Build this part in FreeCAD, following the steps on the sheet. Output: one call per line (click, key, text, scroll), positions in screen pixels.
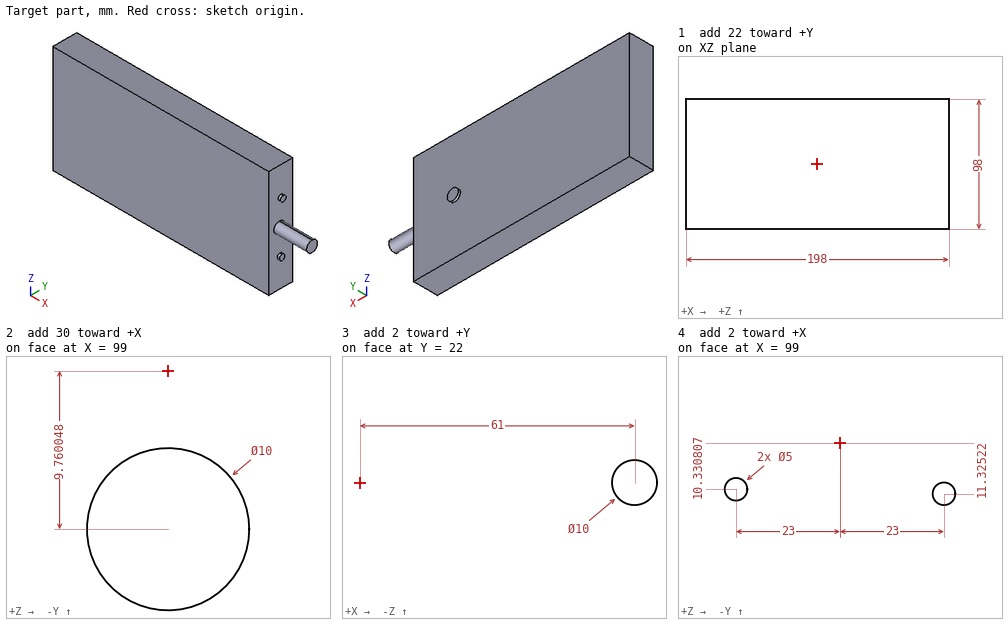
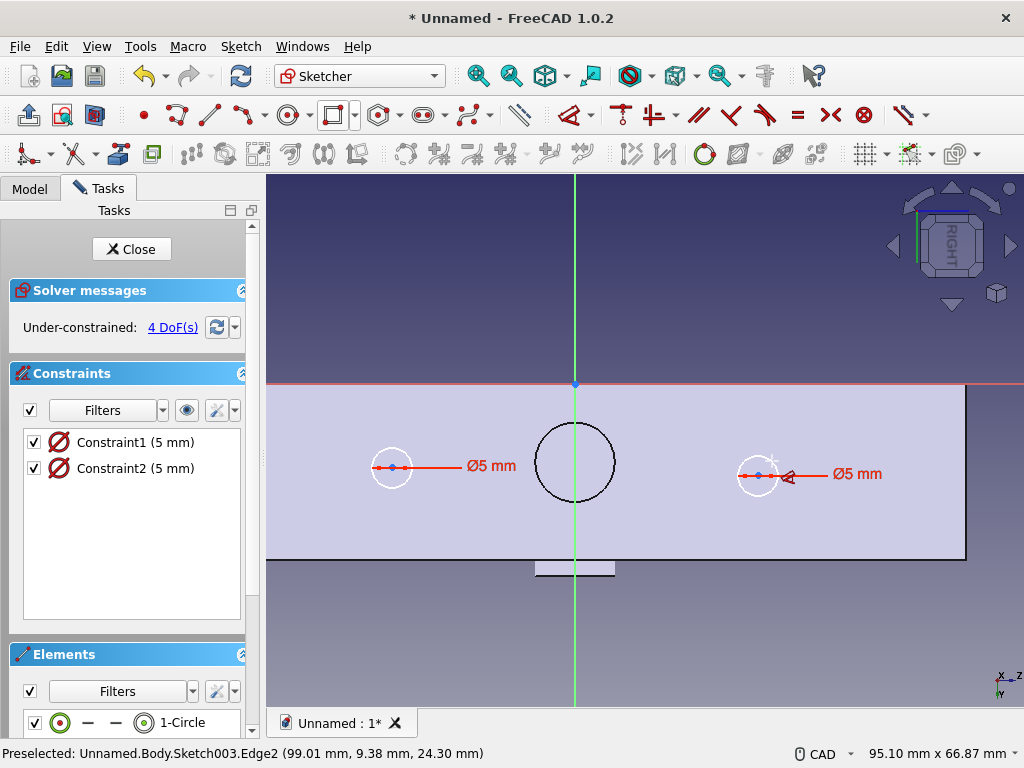
click(392, 468)
click(484, 350)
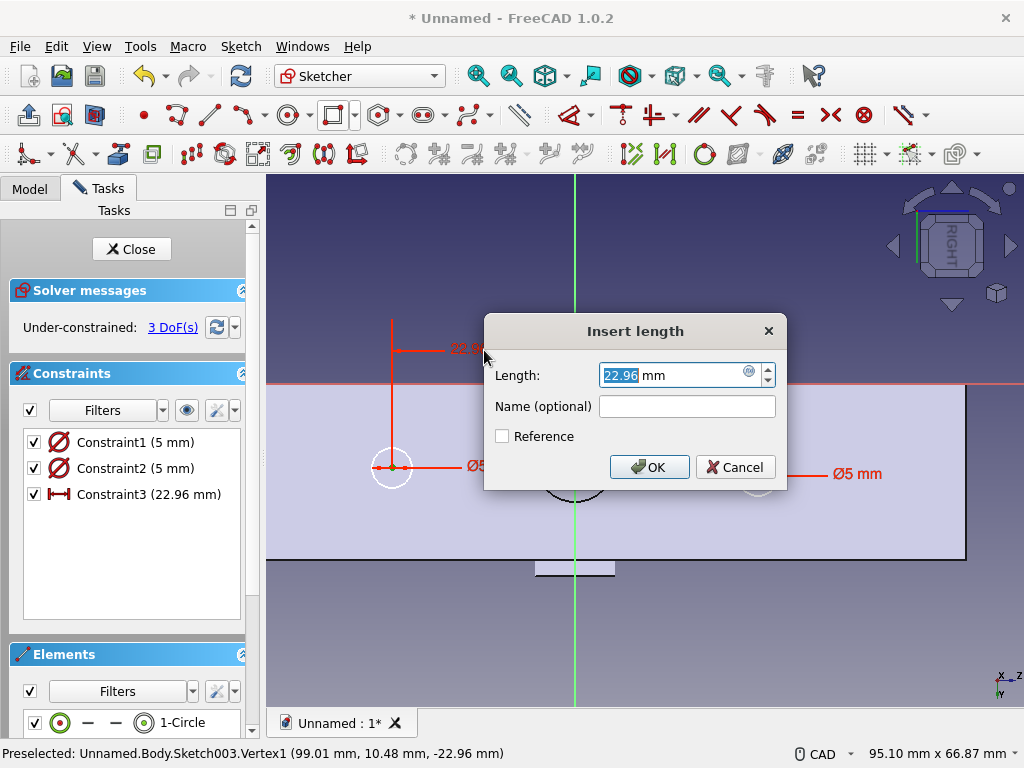
text(23)
key(Return)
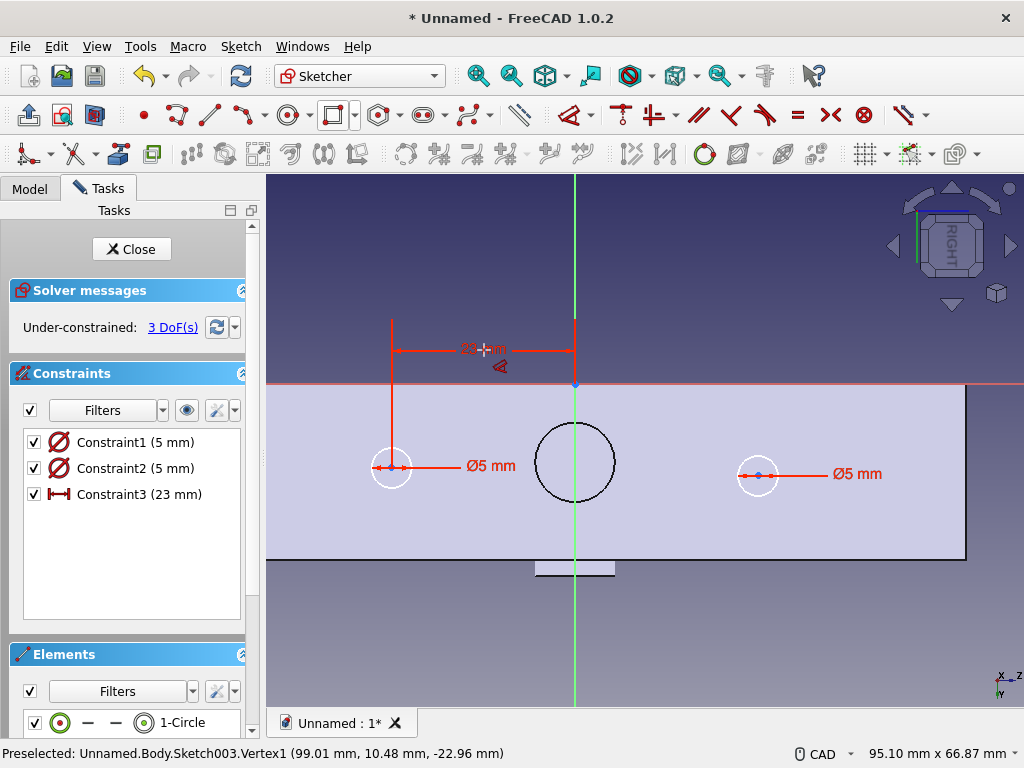
click(758, 476)
click(667, 350)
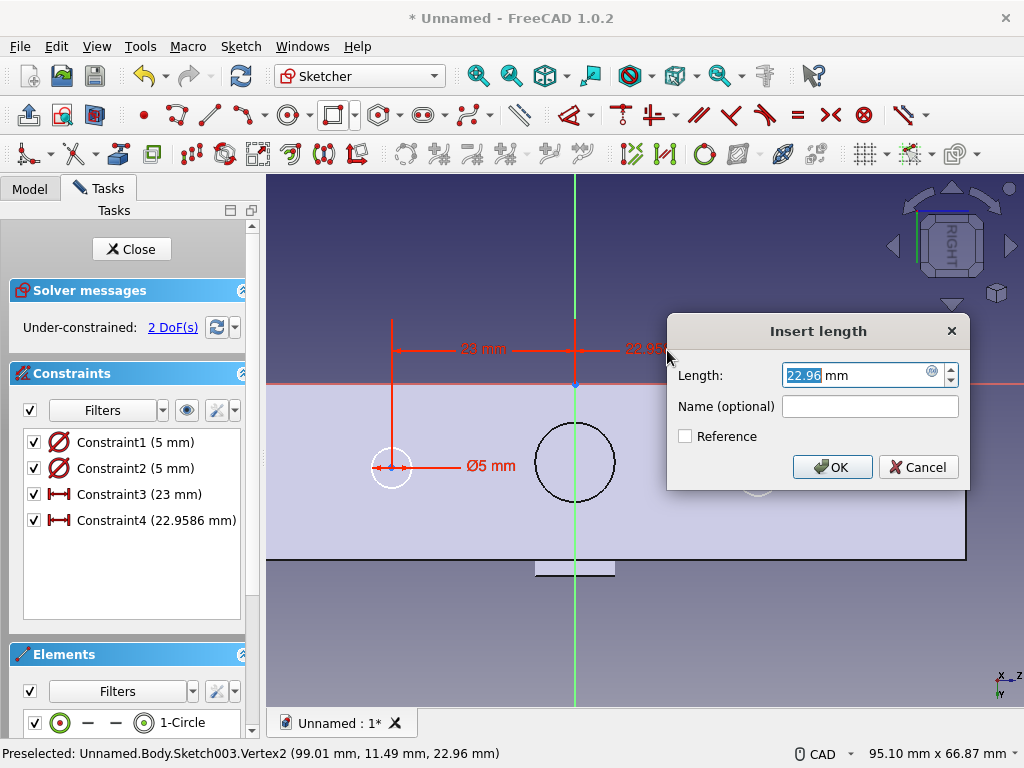
text(23)
key(Return)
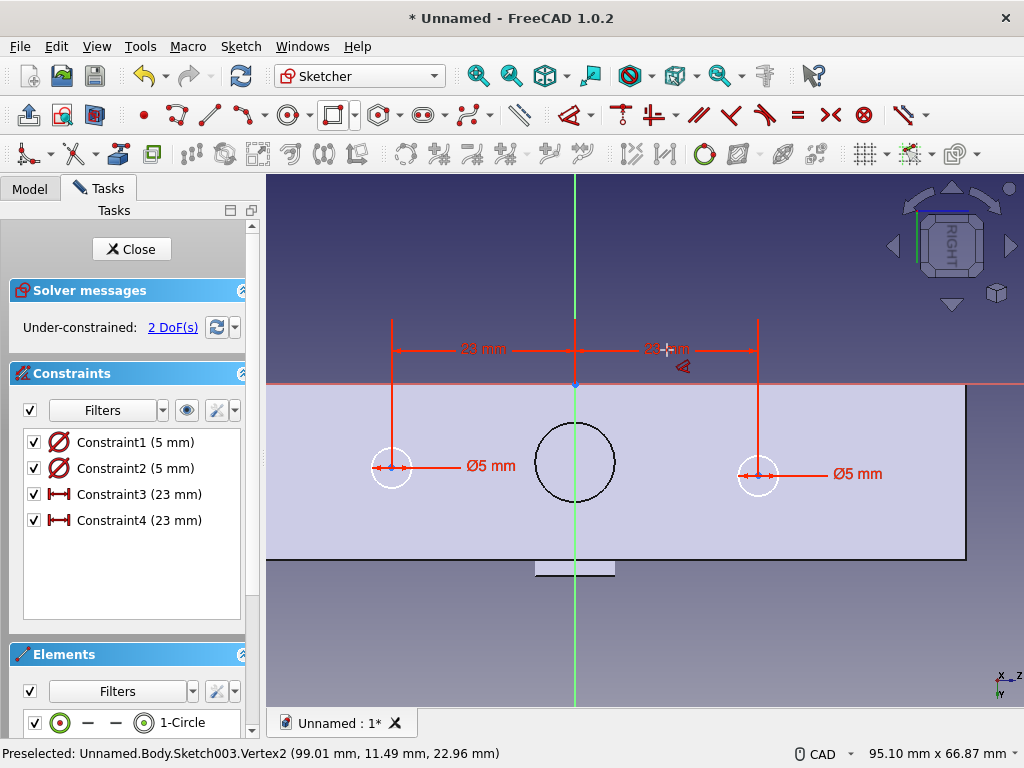
click(758, 476)
click(792, 430)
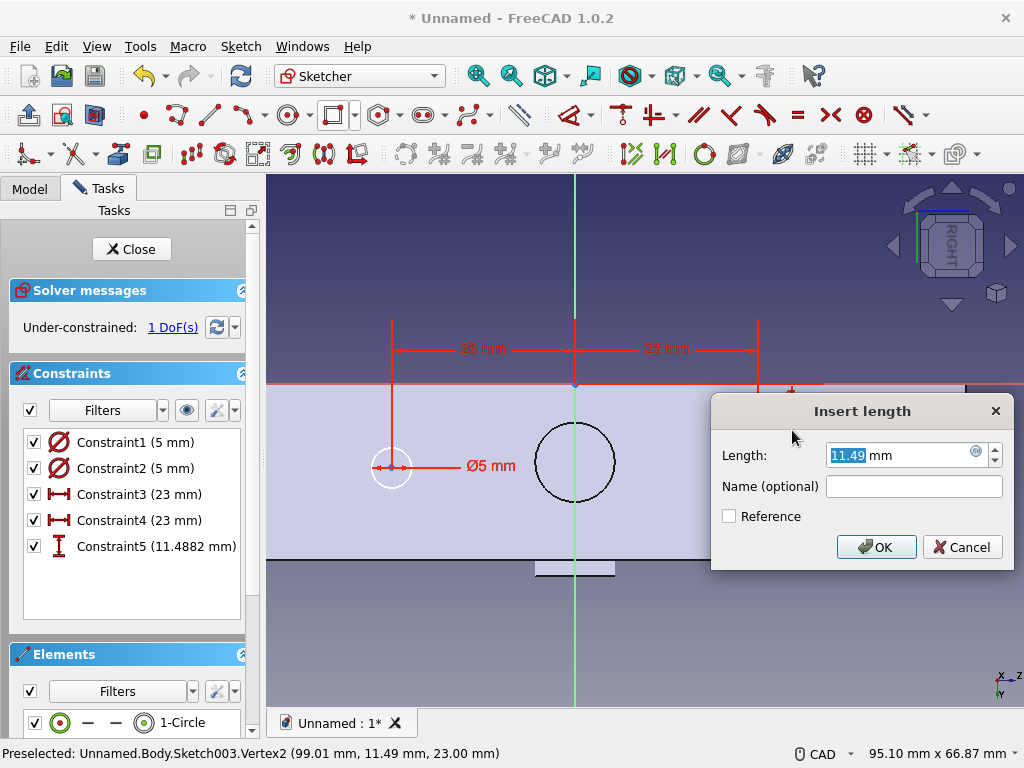
text(11.32522)
key(Return)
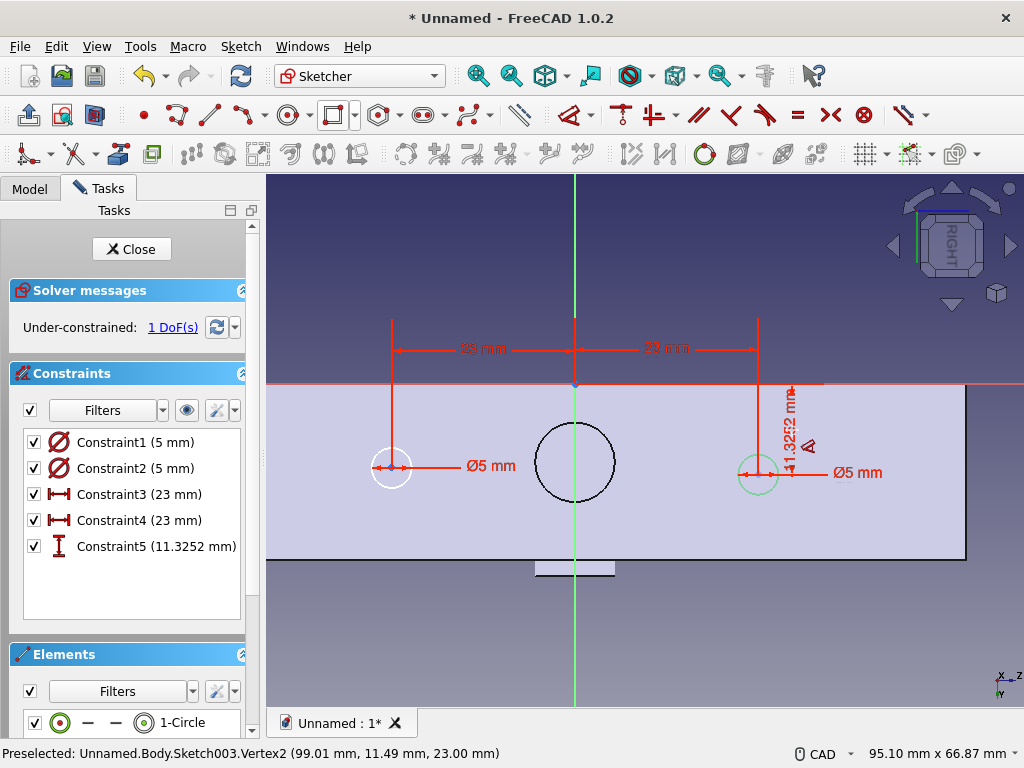
click(392, 468)
click(358, 426)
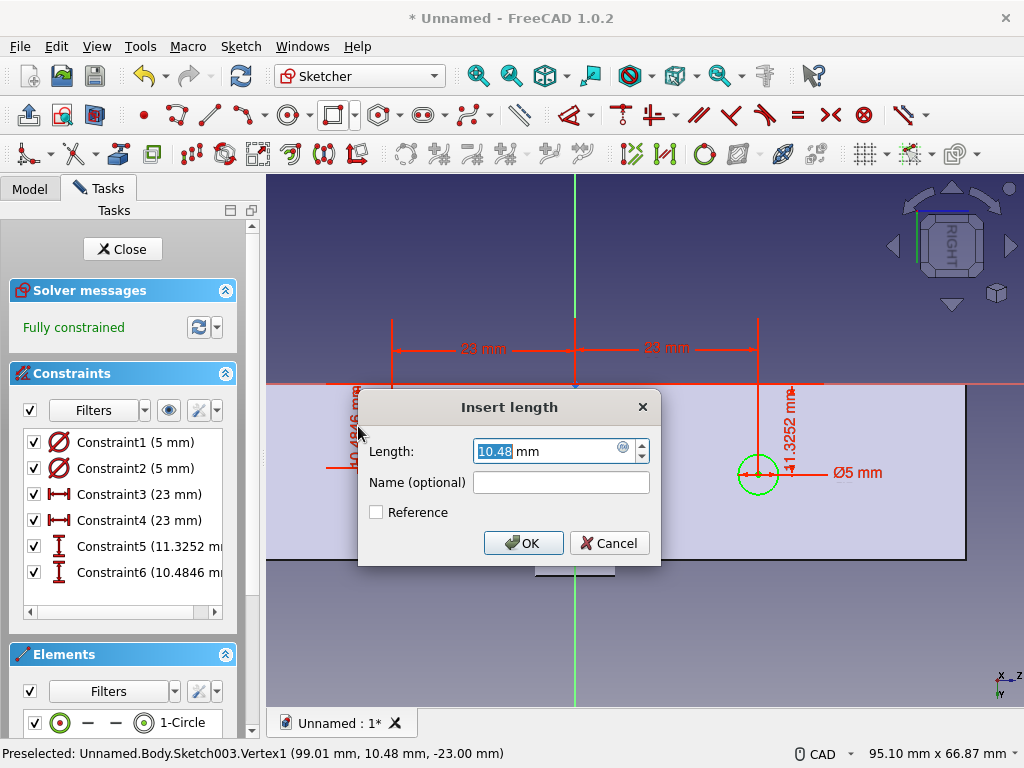
text(10.330807)
key(Return)
key(Escape)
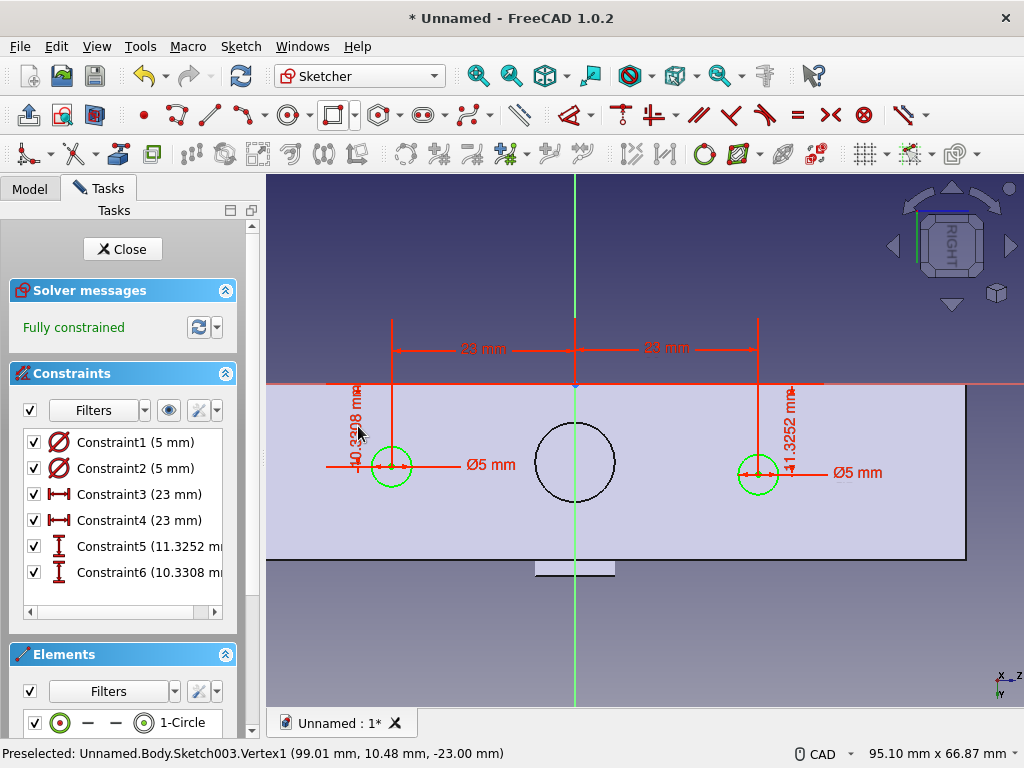
click(123, 249)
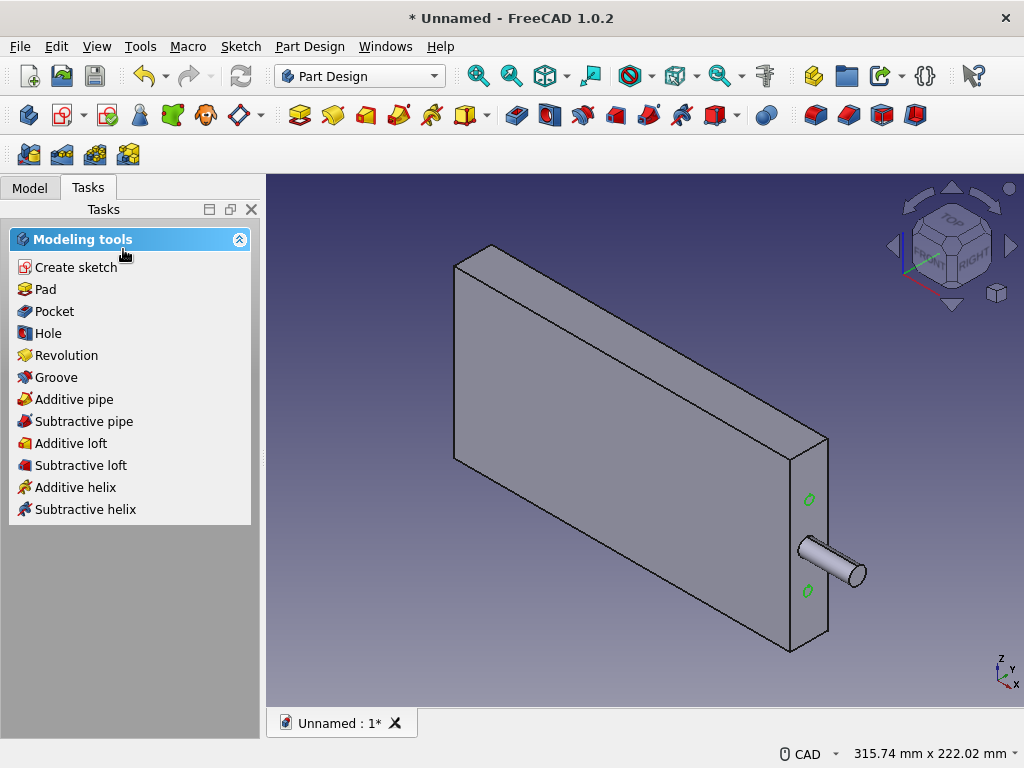
click(300, 116)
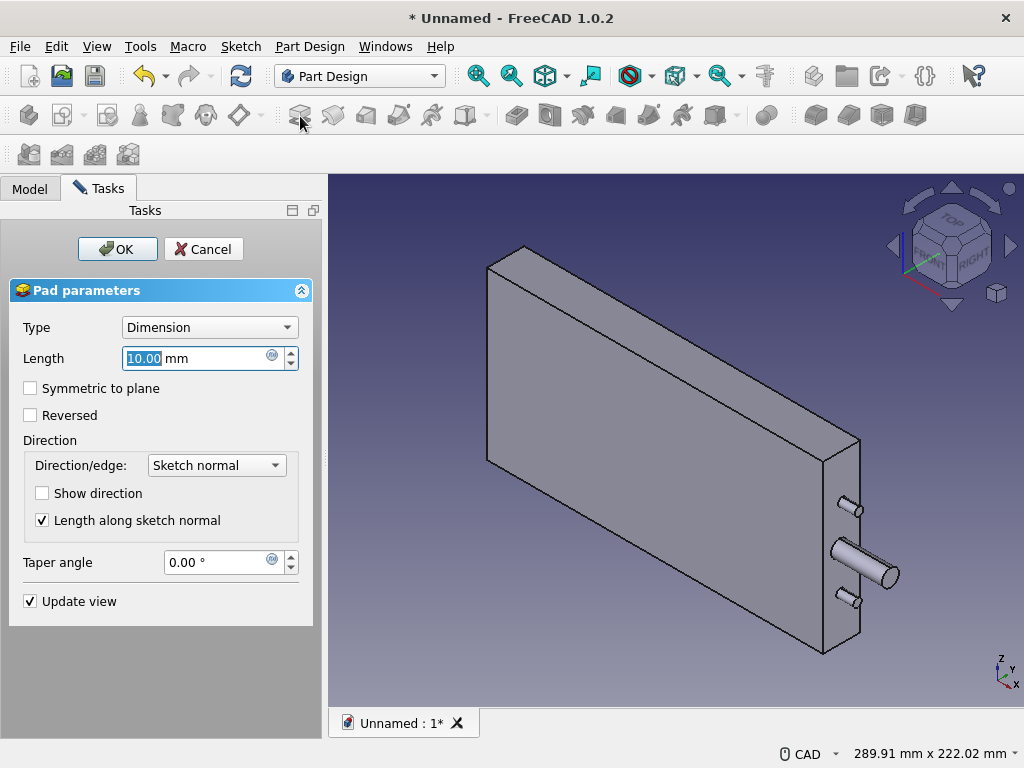
text(2)
key(Tab)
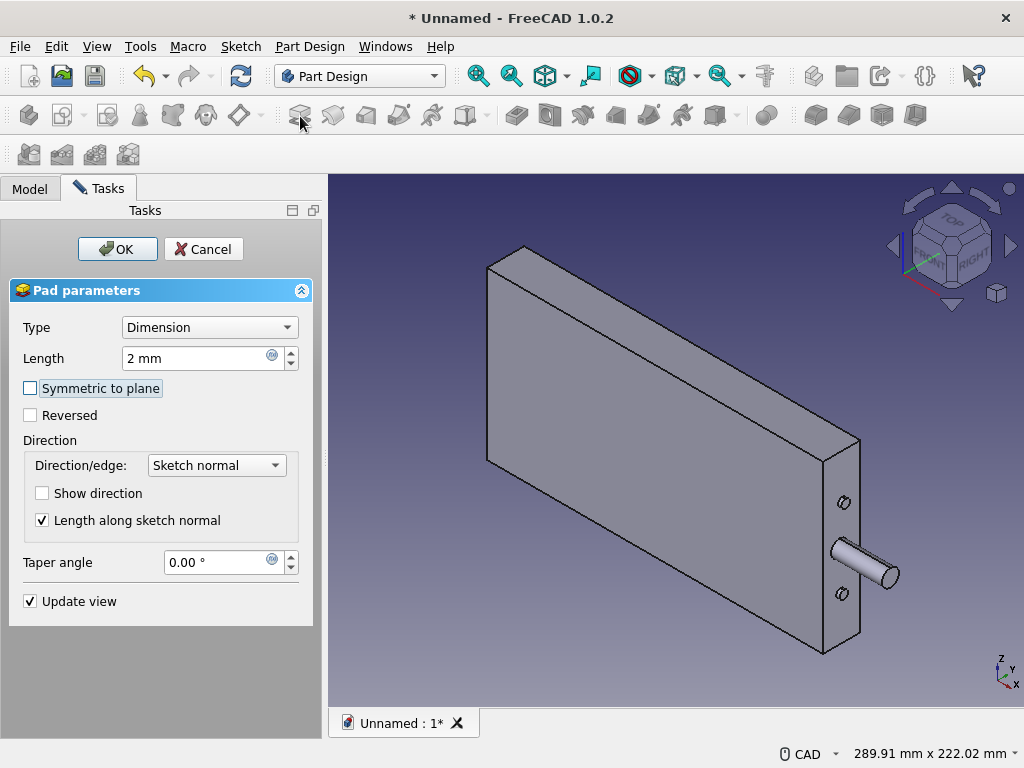
click(118, 249)